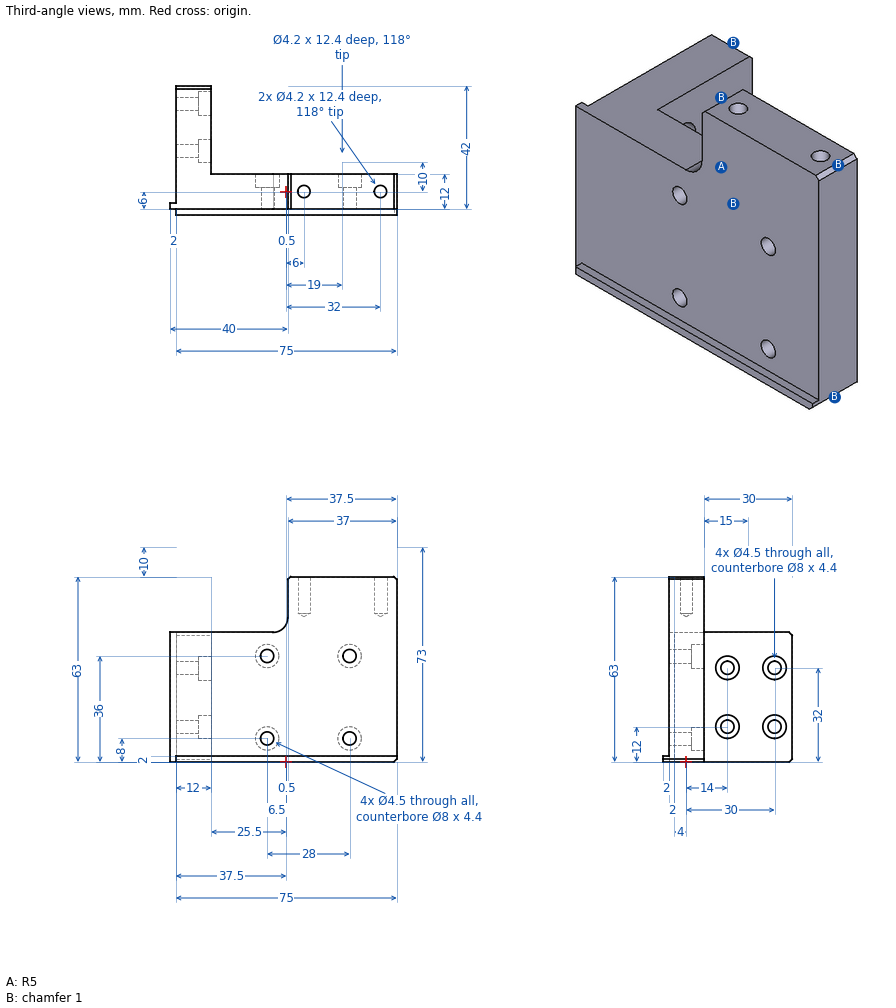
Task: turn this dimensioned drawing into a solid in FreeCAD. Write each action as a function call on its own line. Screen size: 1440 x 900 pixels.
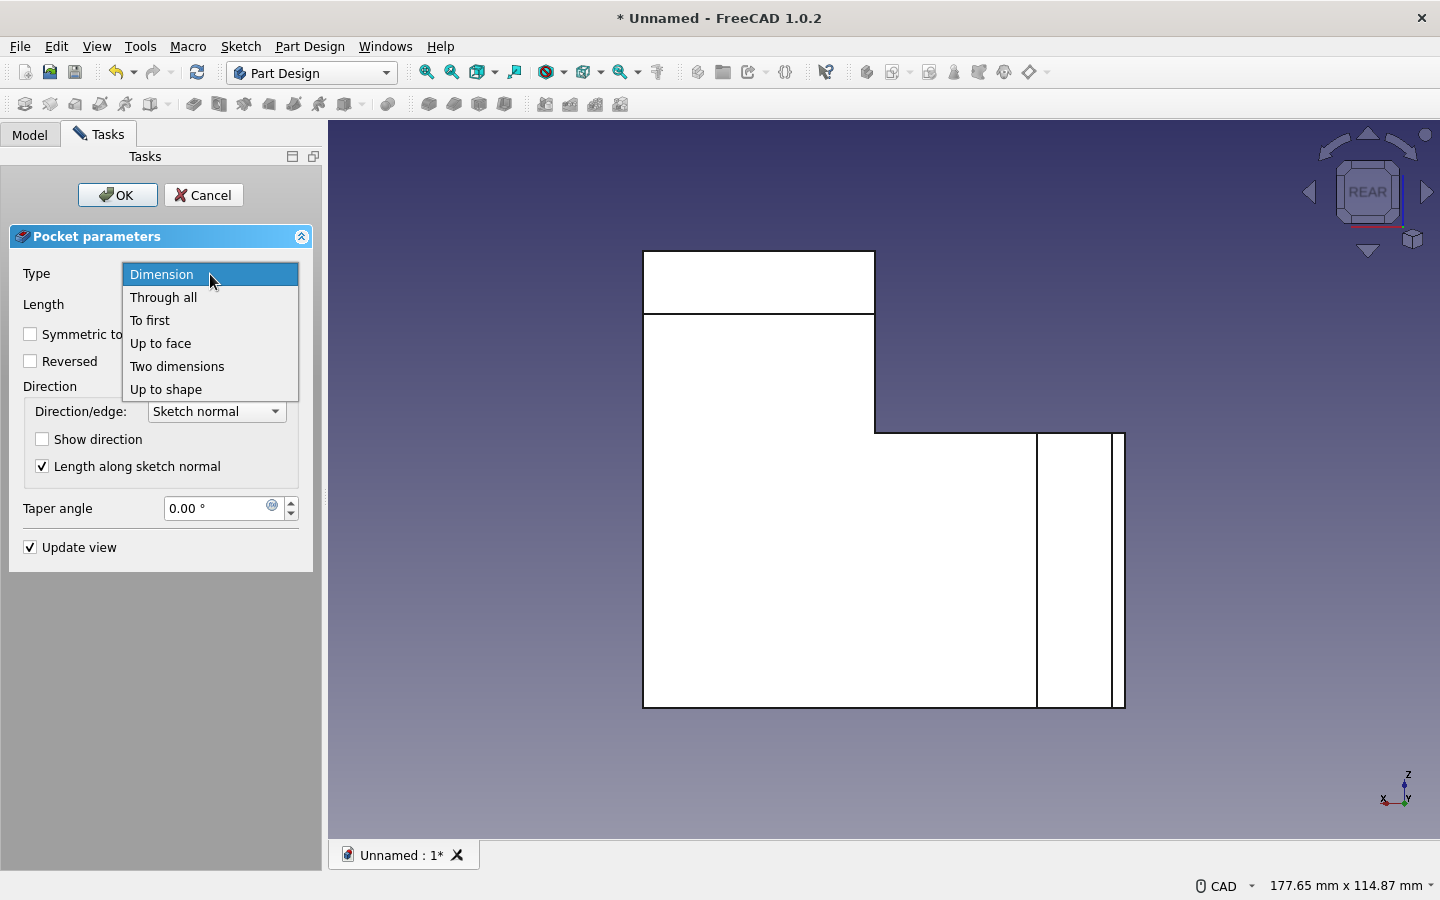
click(208, 298)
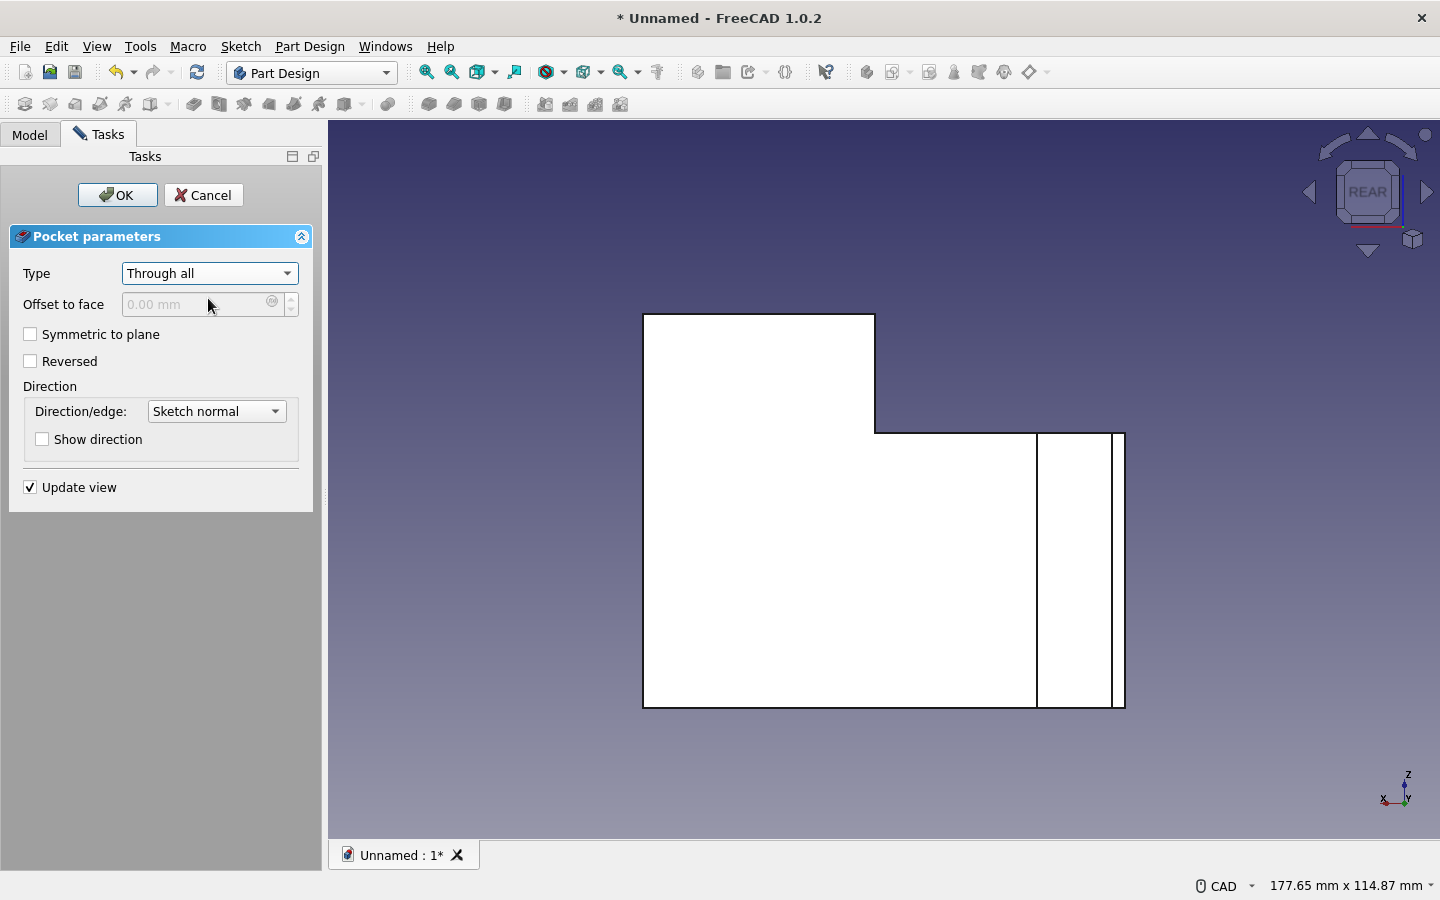
click(118, 195)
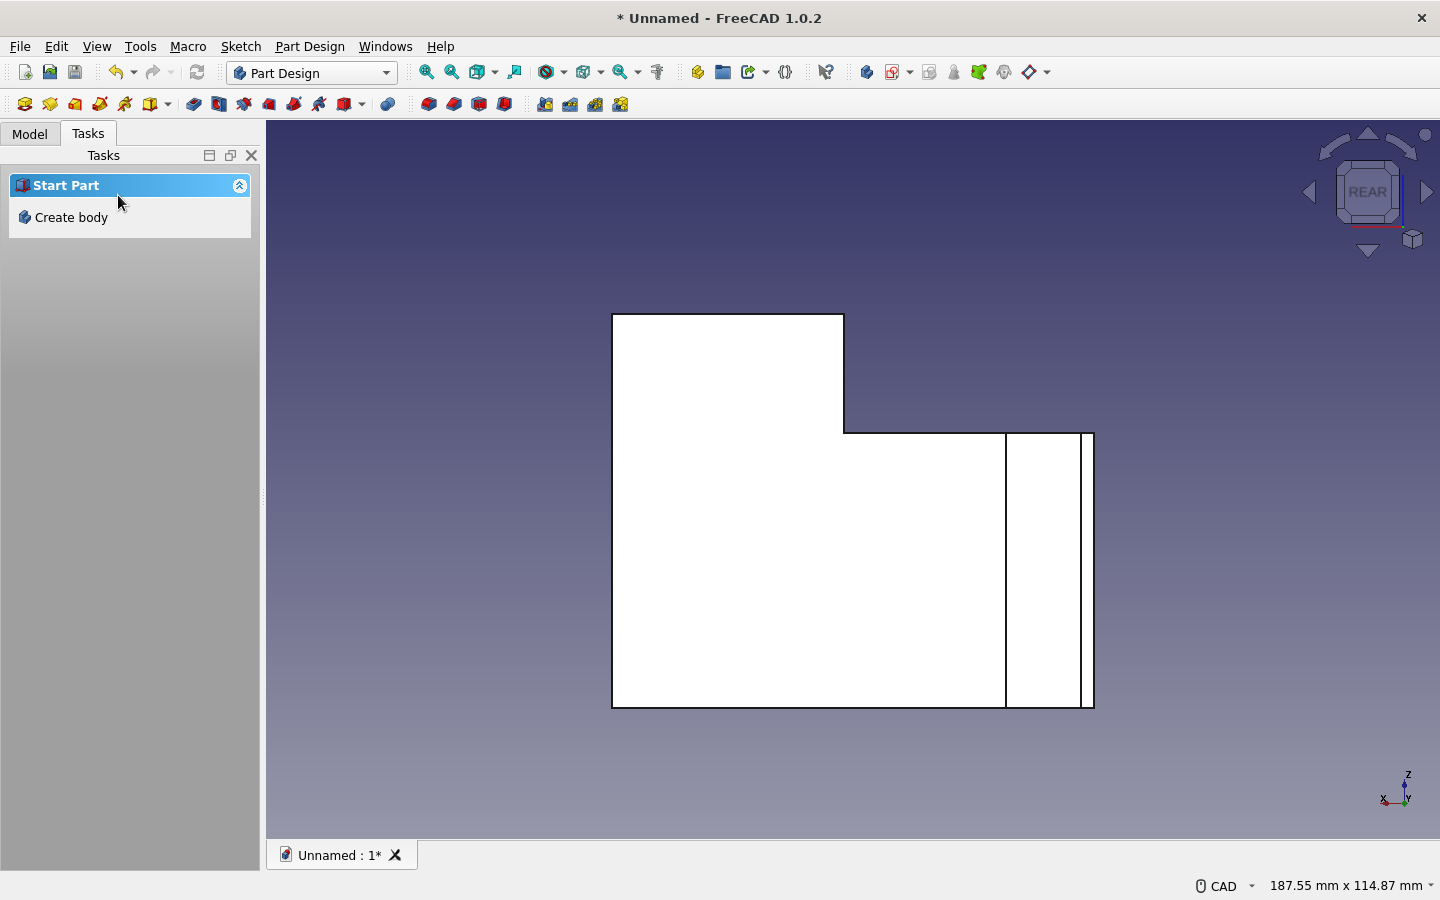
key(0)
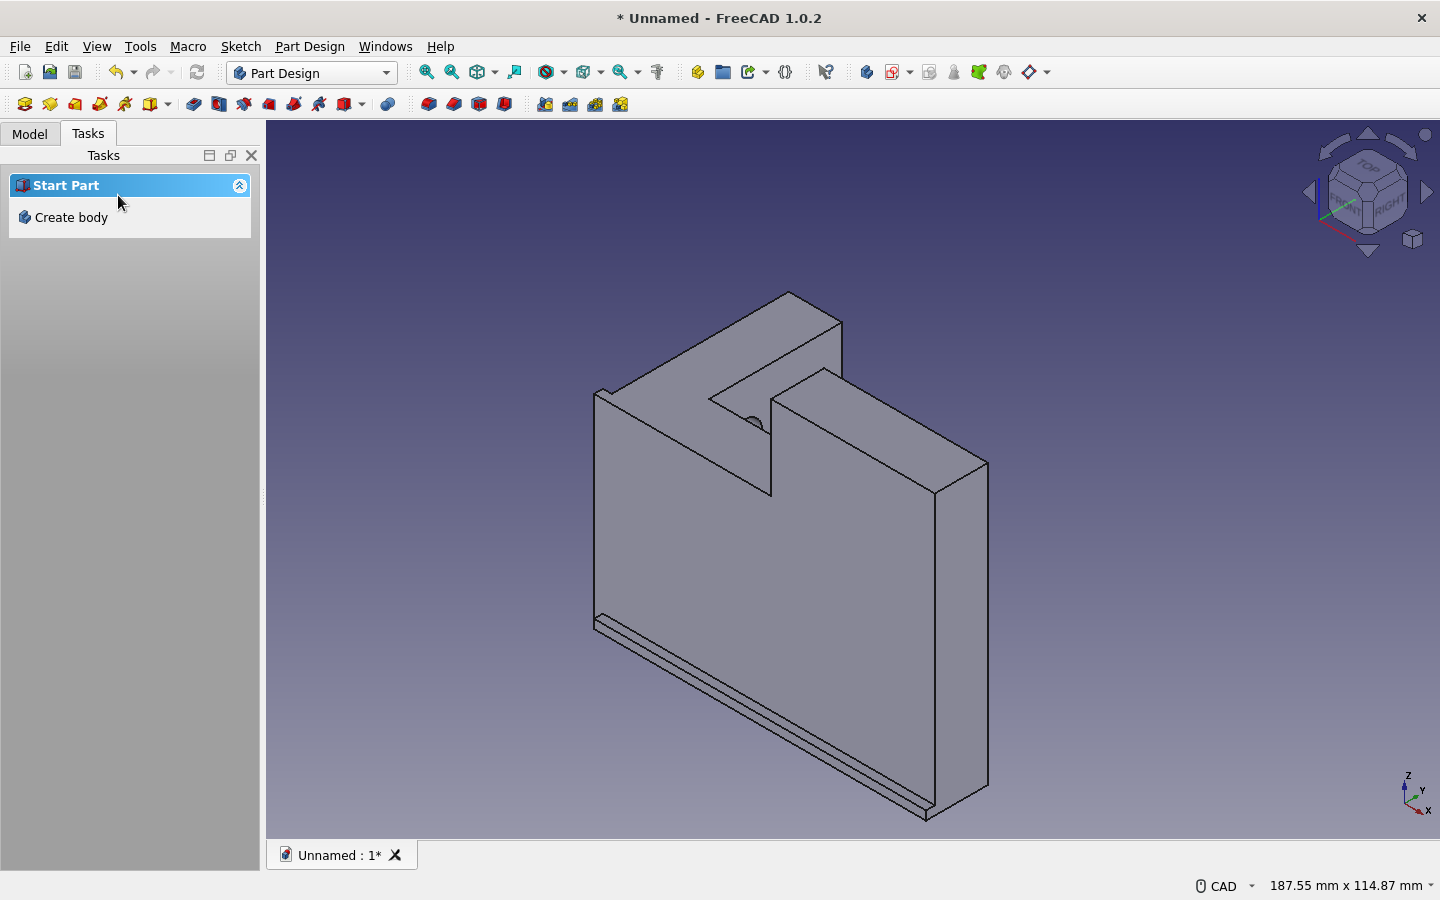
click(926, 457)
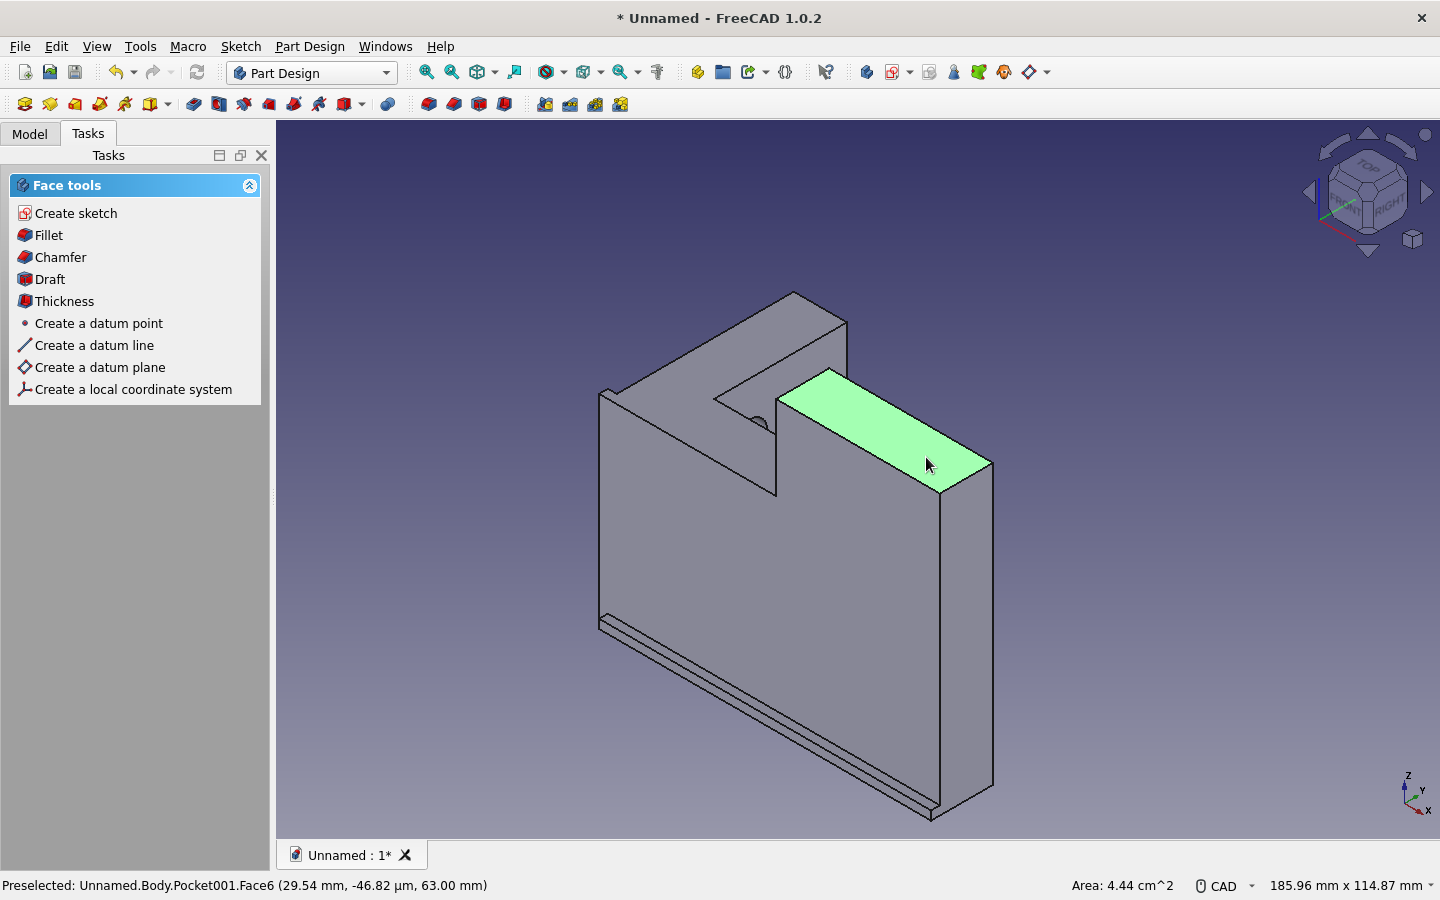
click(892, 72)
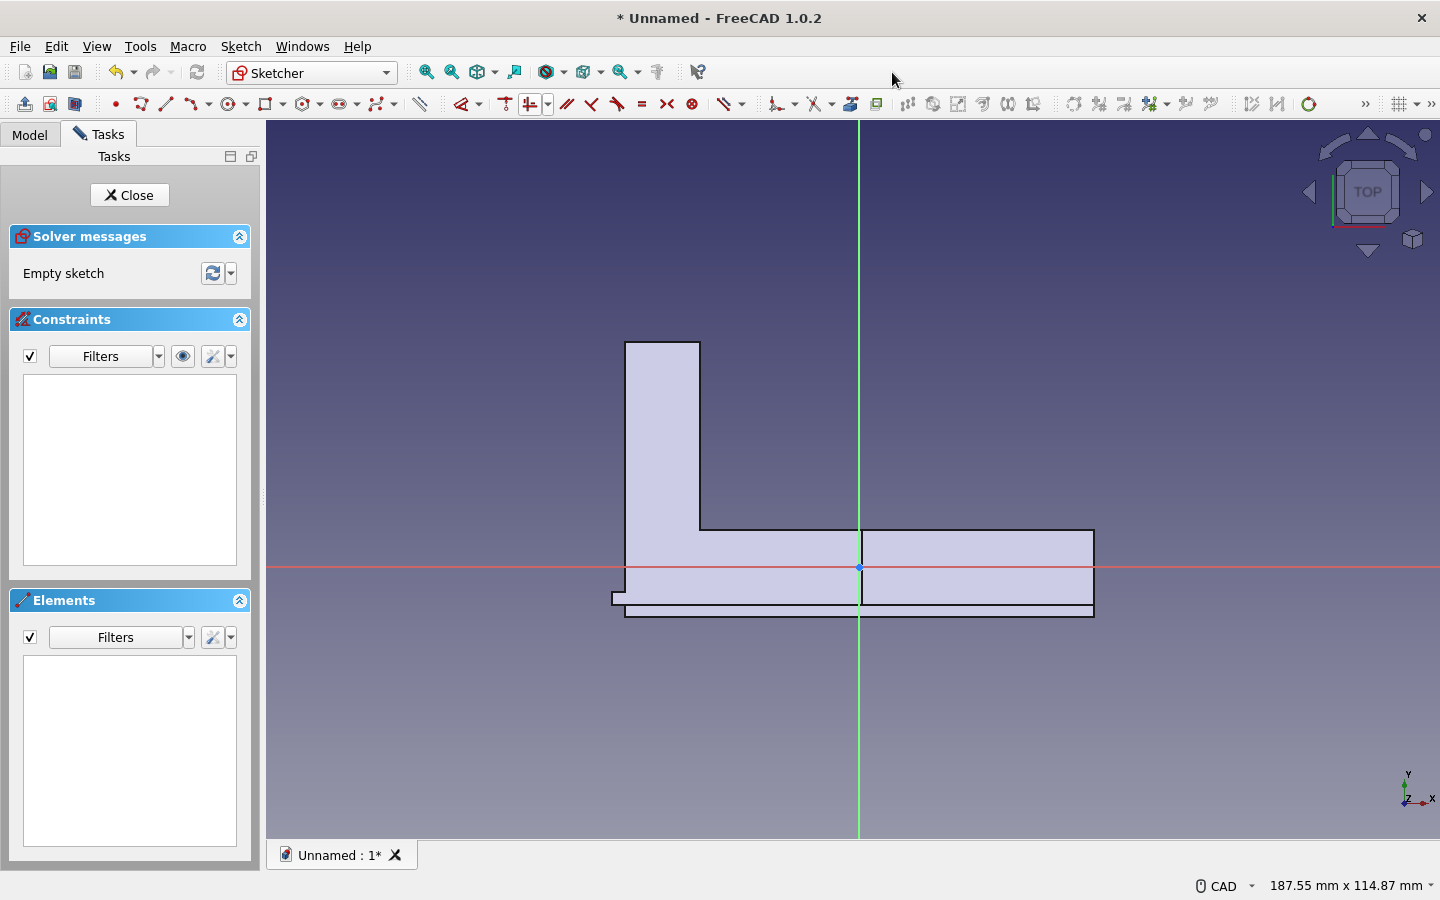
scroll(1044, 605, up, 6)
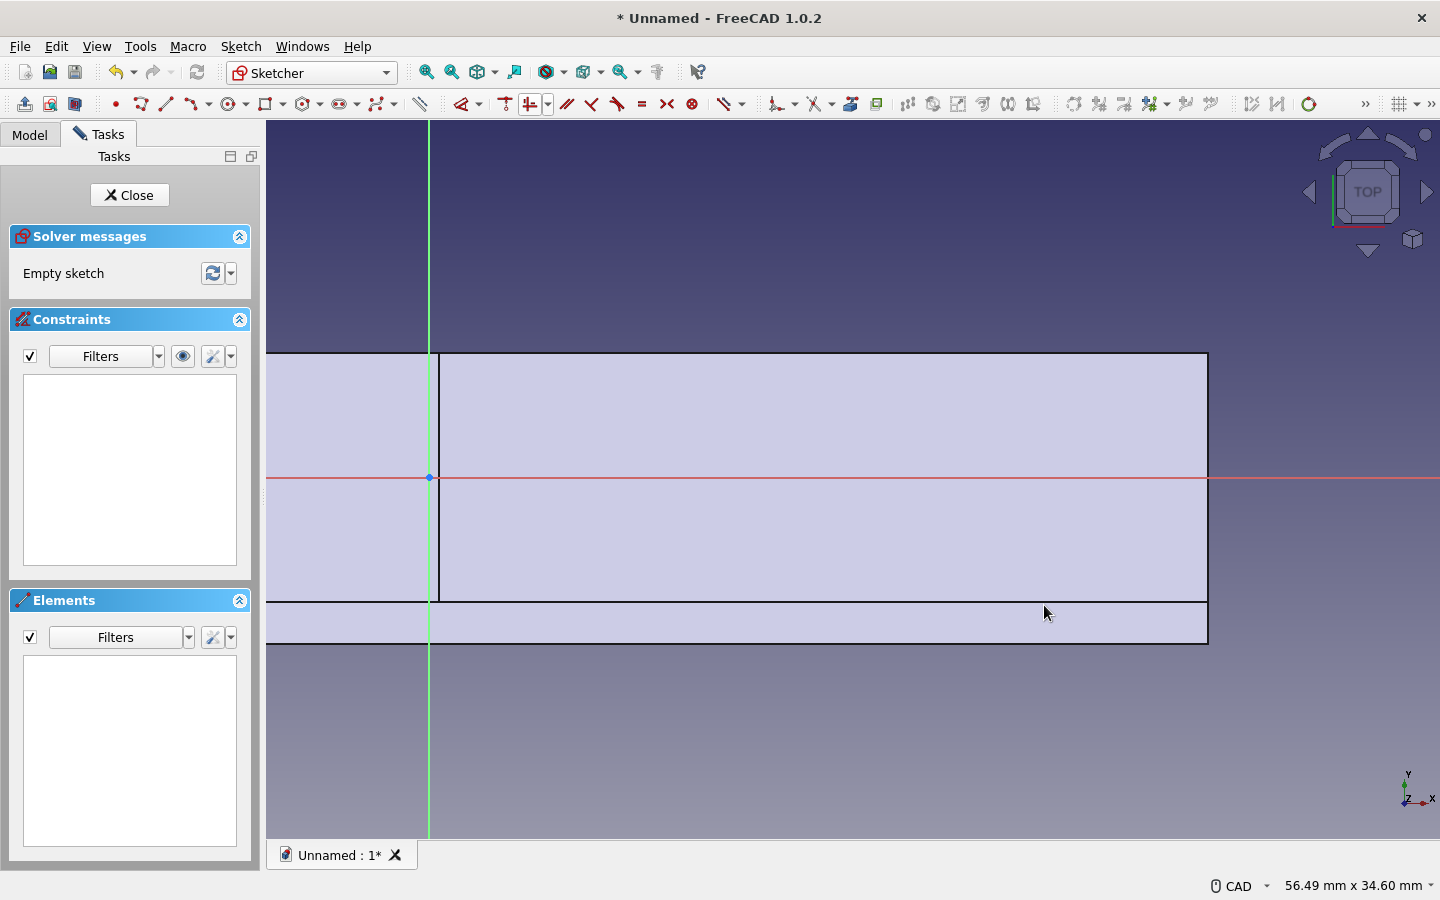
click(228, 104)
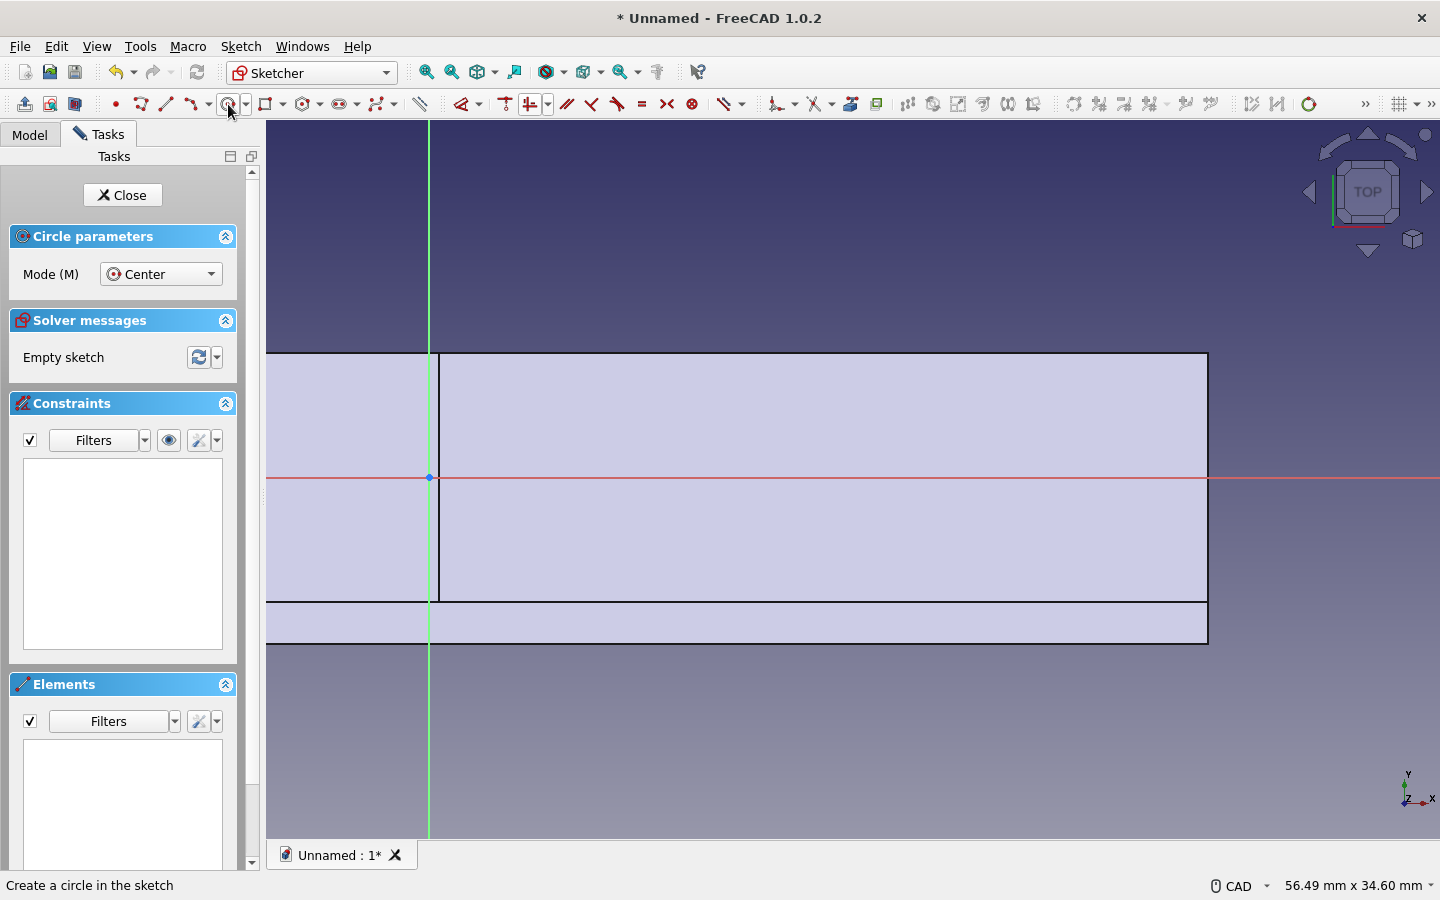
click(1094, 478)
move(1125, 447)